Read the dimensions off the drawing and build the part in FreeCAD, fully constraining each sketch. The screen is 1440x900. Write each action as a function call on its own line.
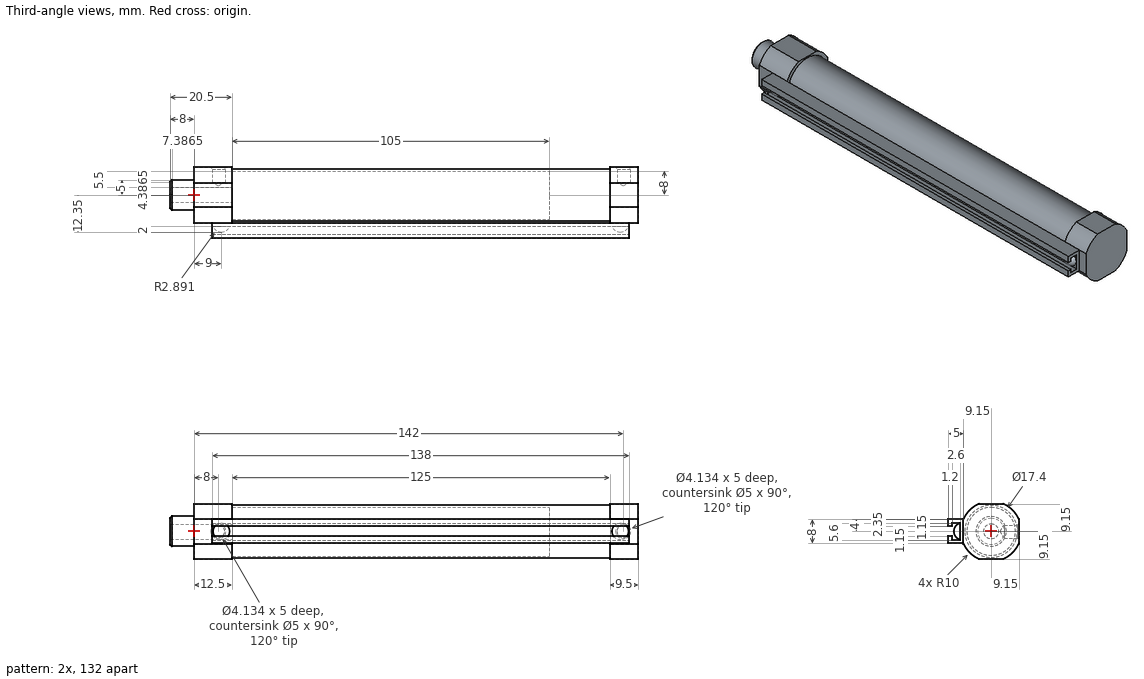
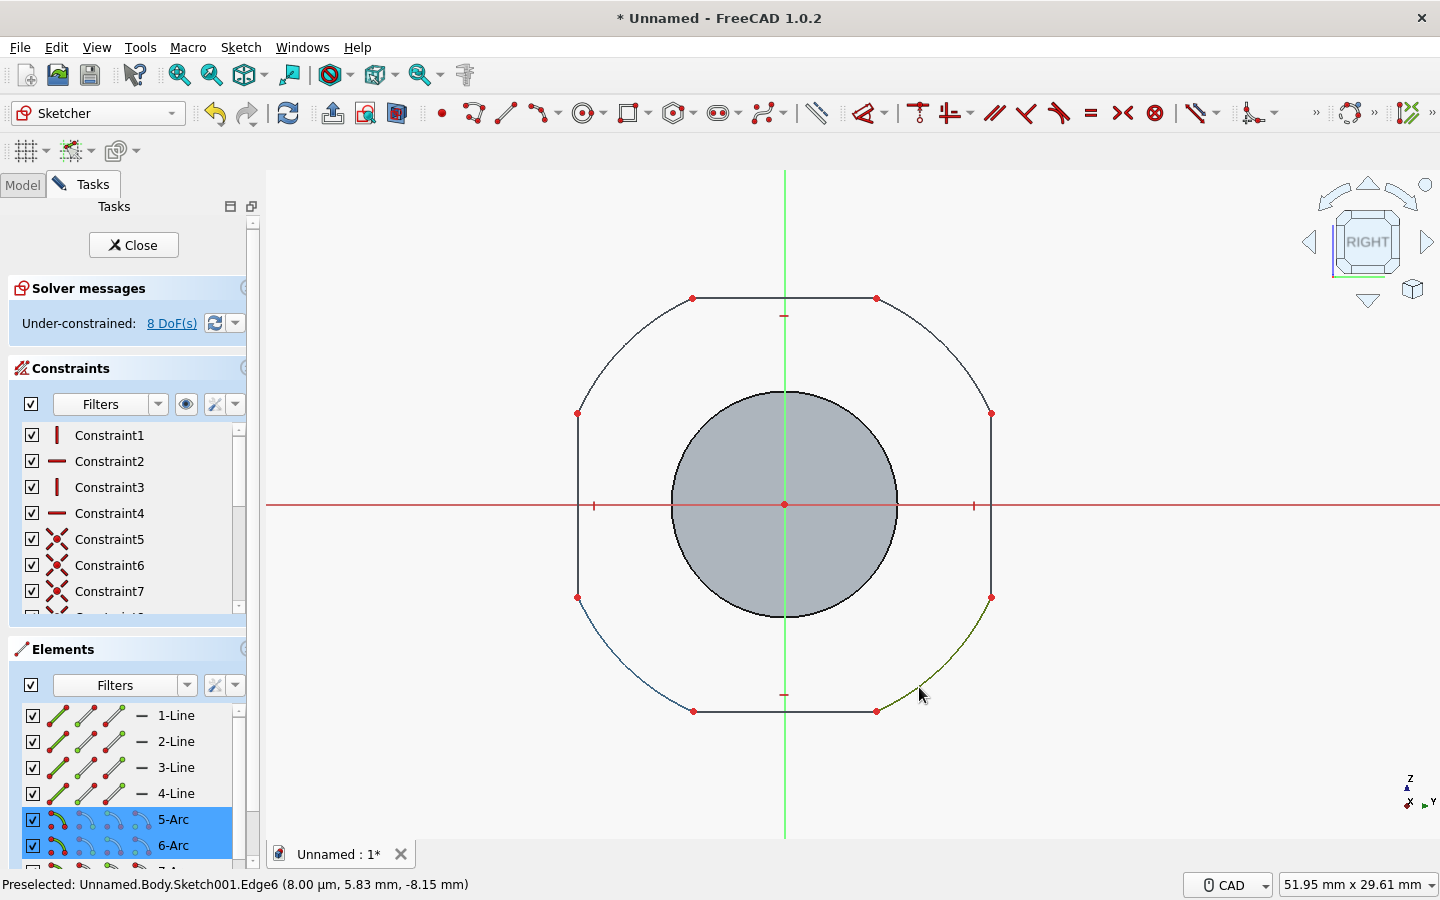
click(966, 371)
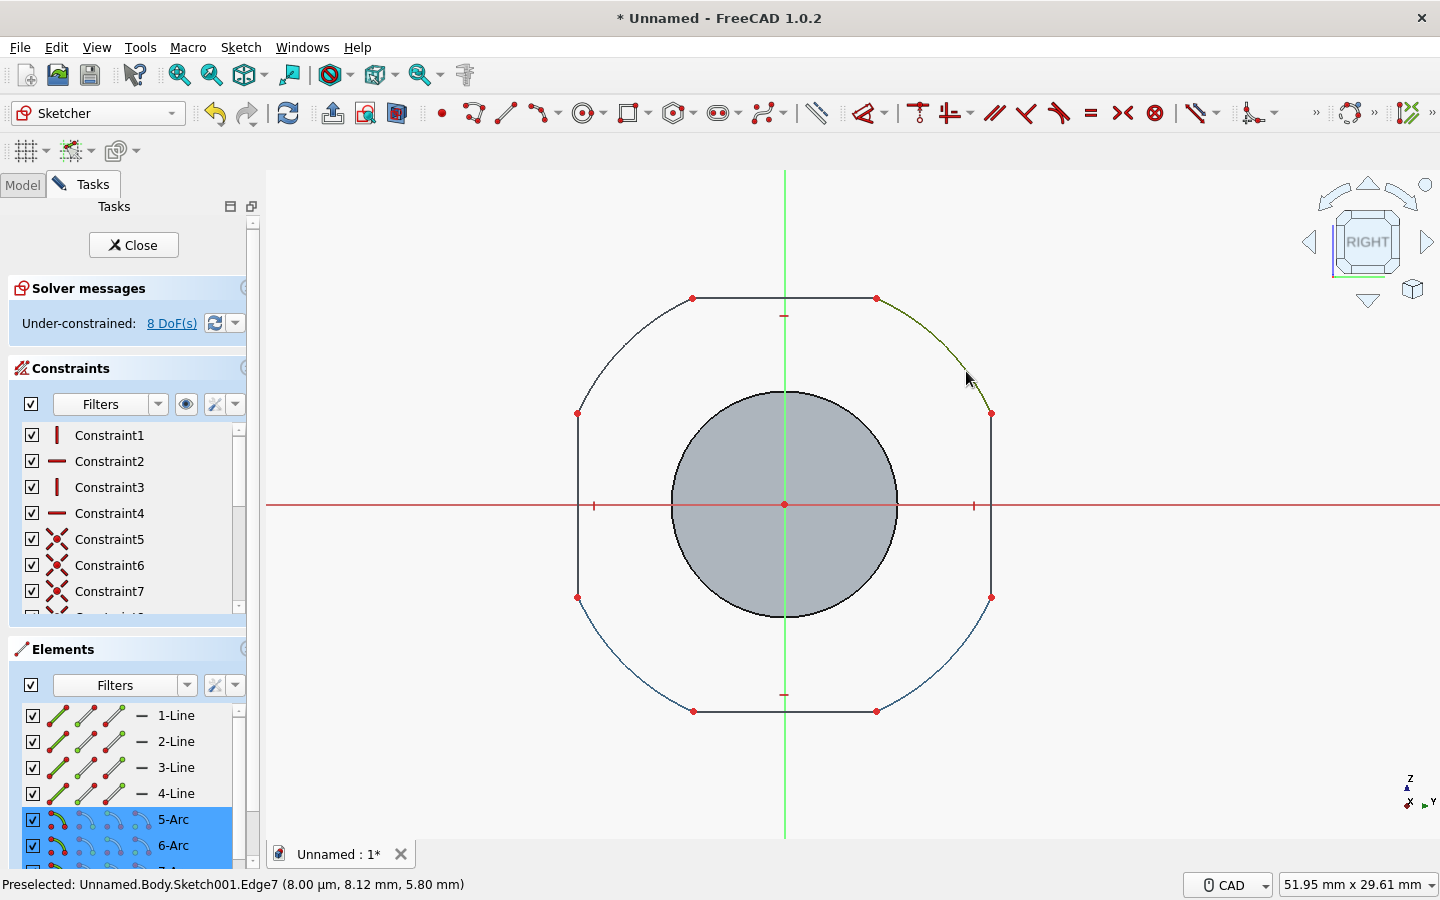
click(650, 324)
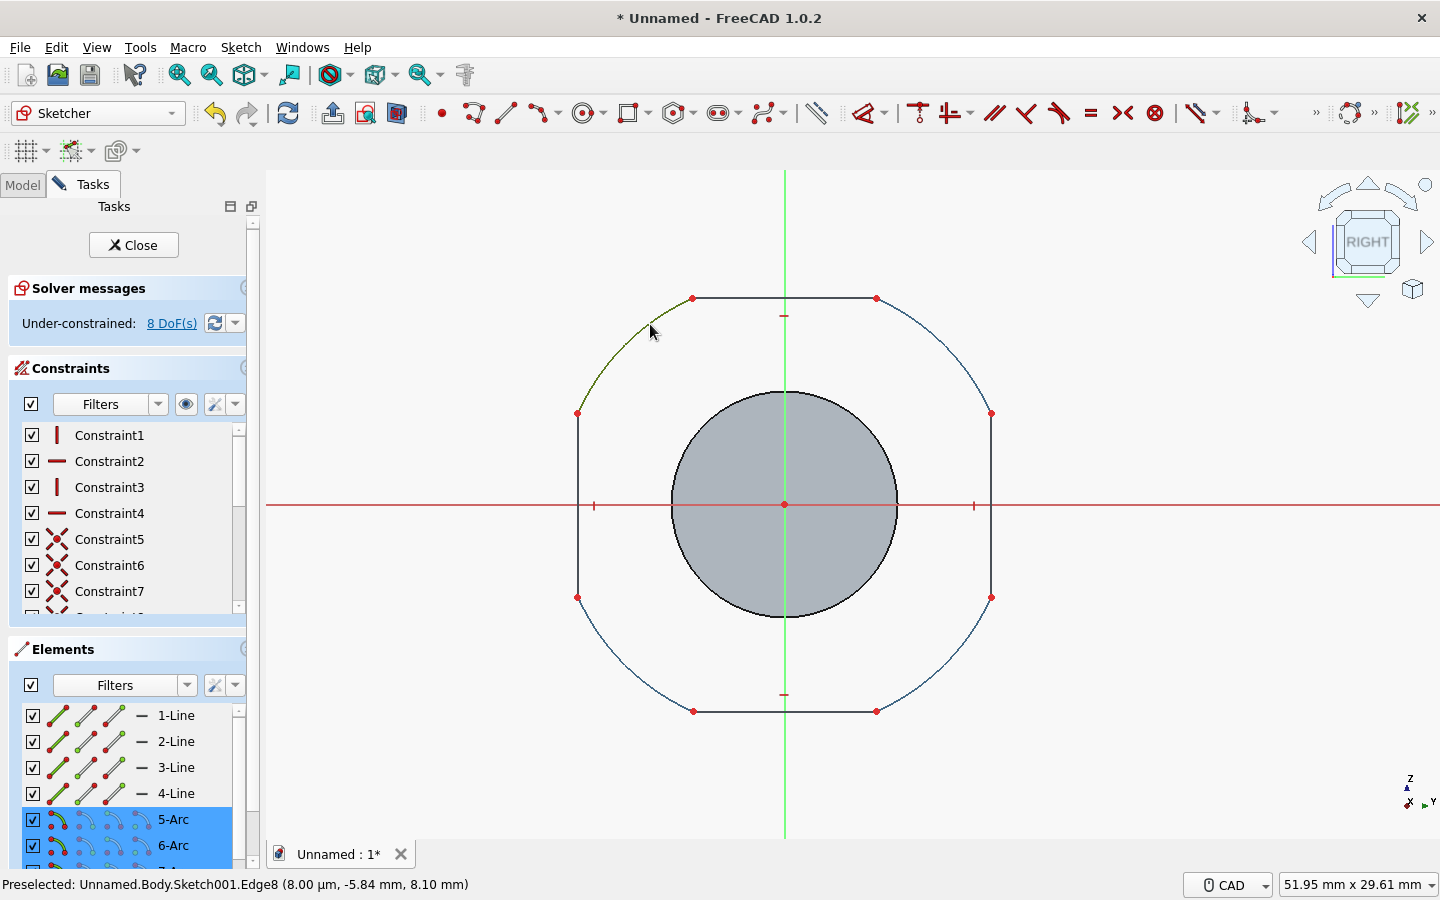
click(1092, 114)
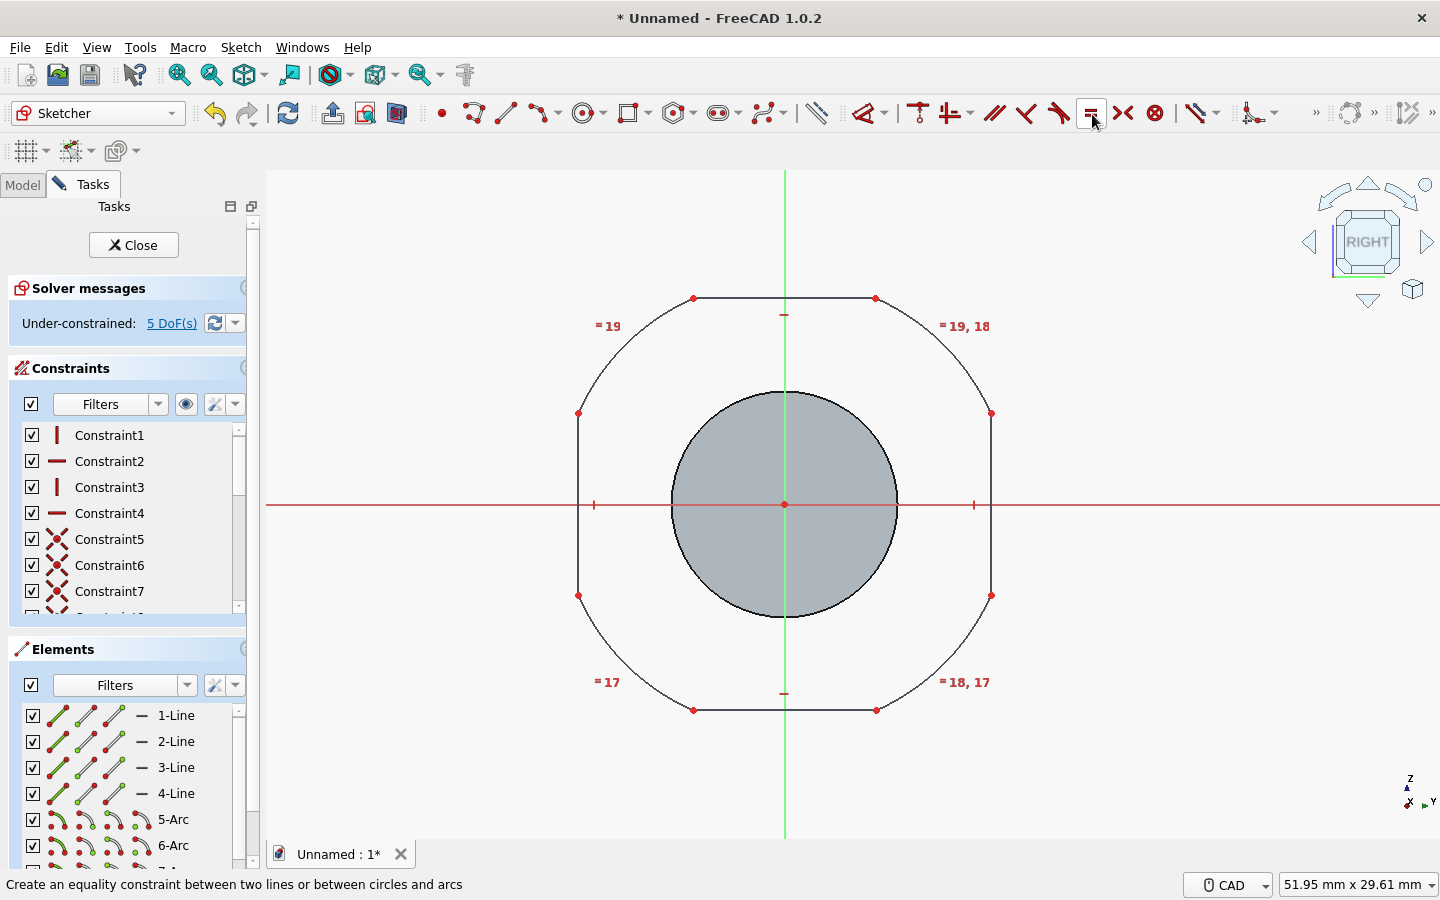
click(864, 114)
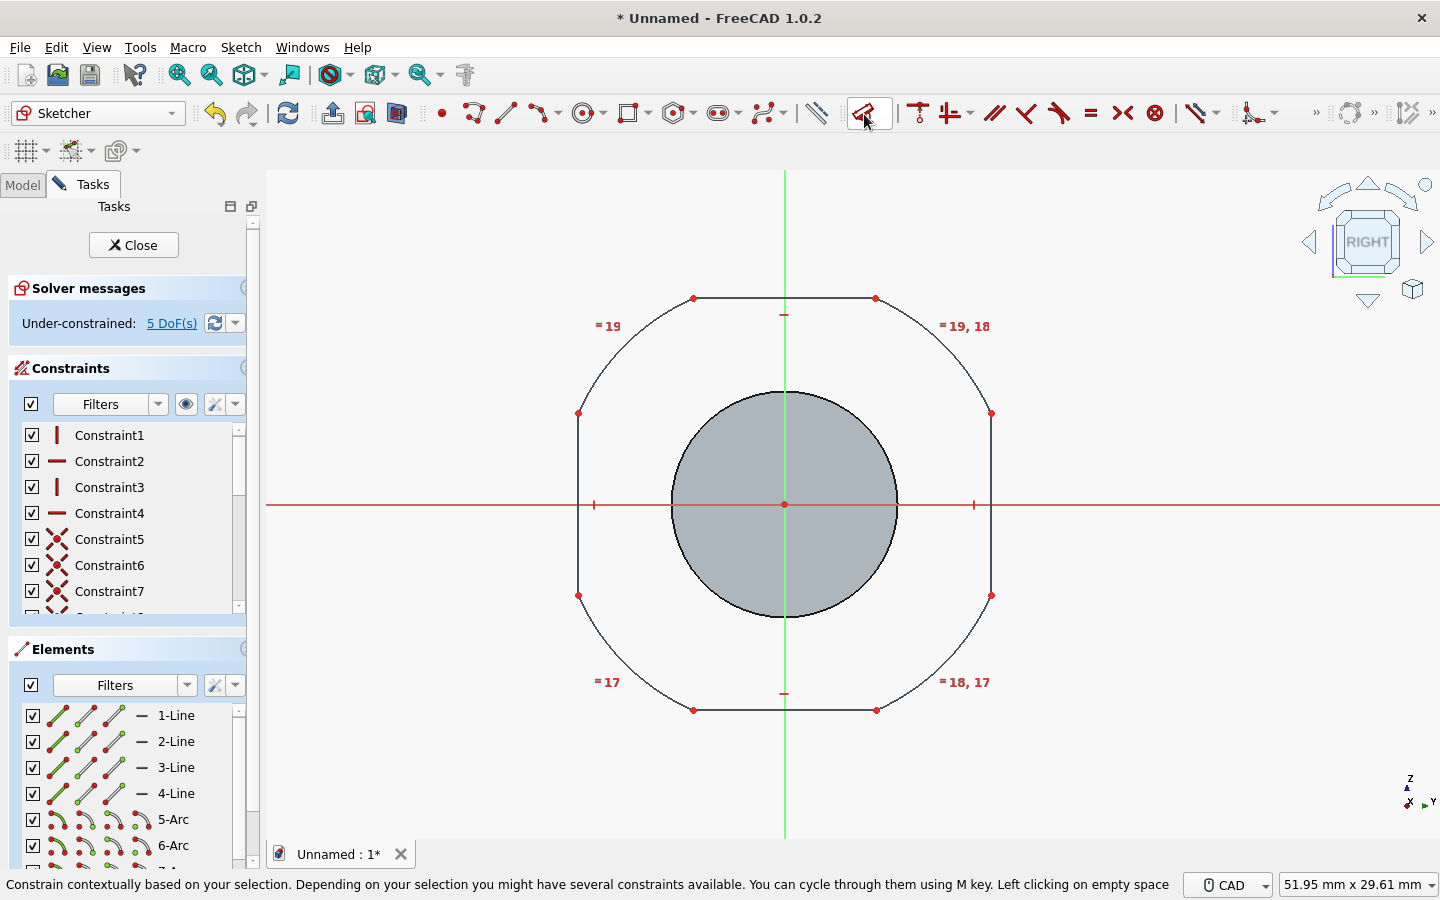
click(603, 638)
click(577, 657)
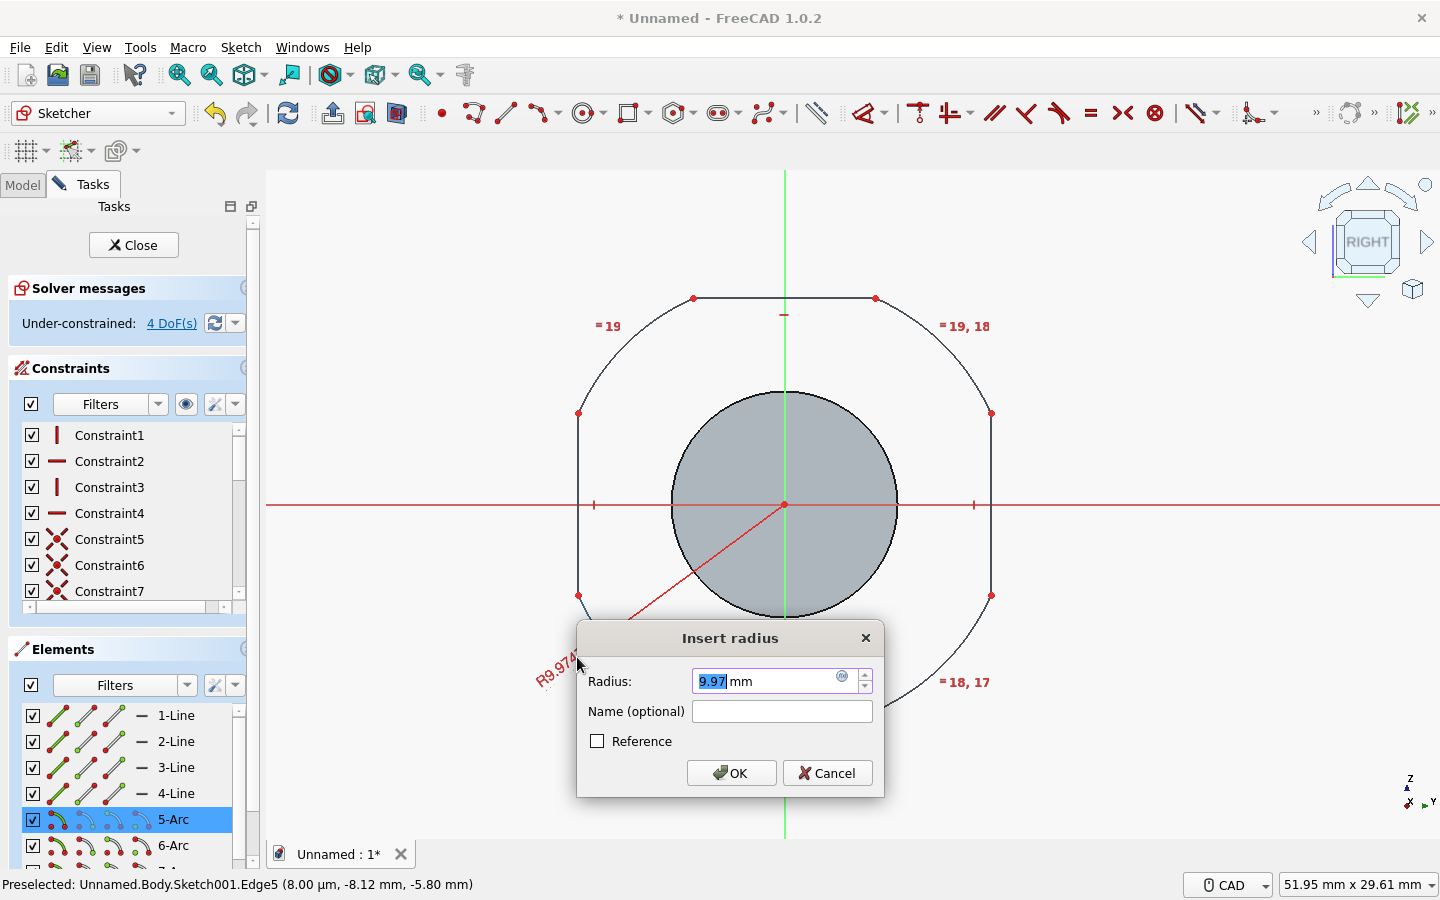
text(10)
key(Return)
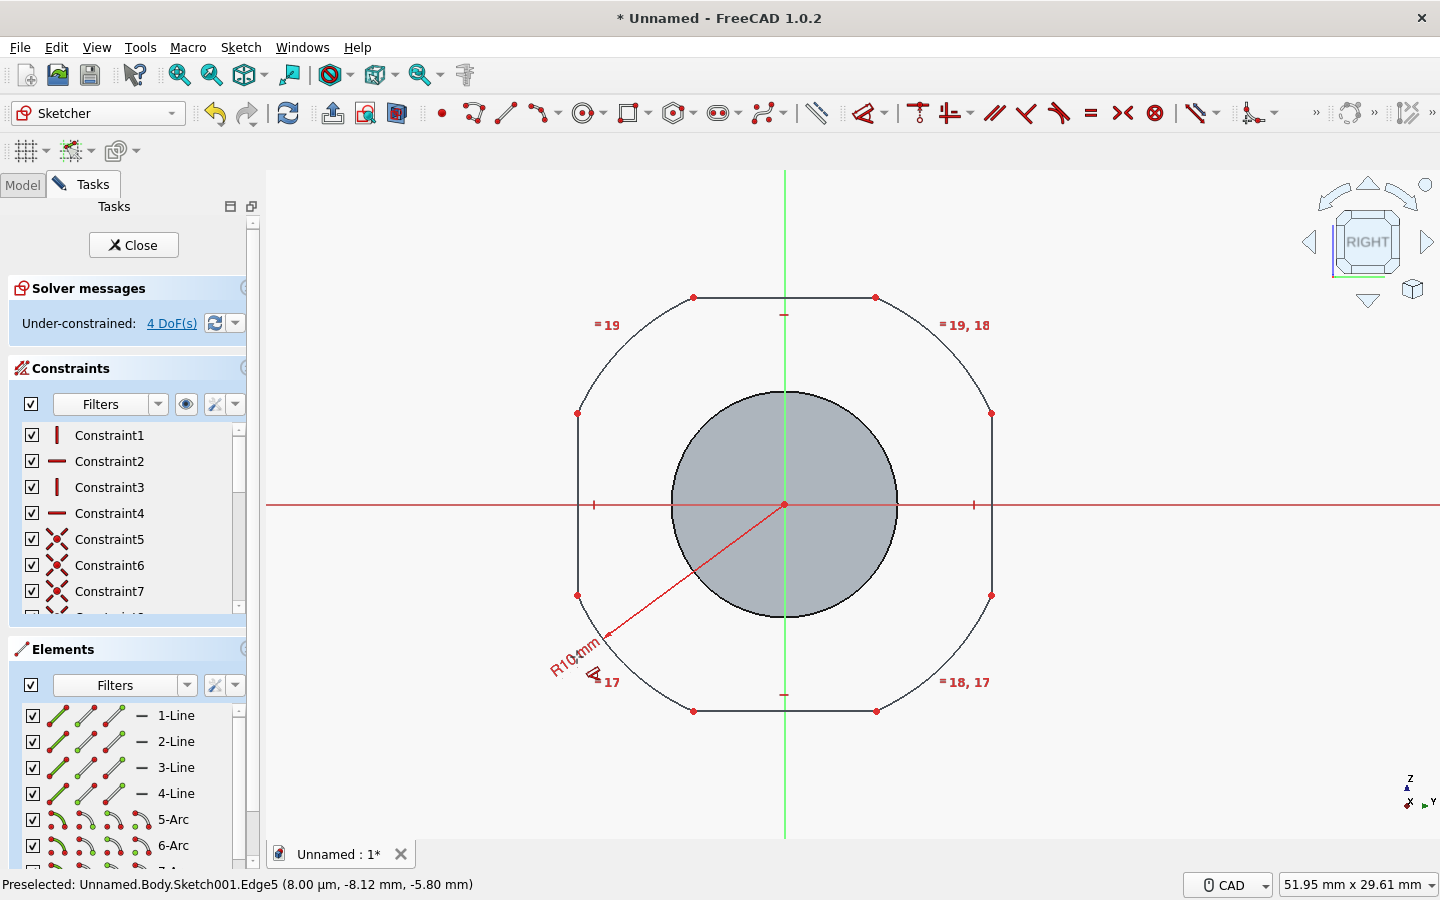
click(578, 414)
click(681, 380)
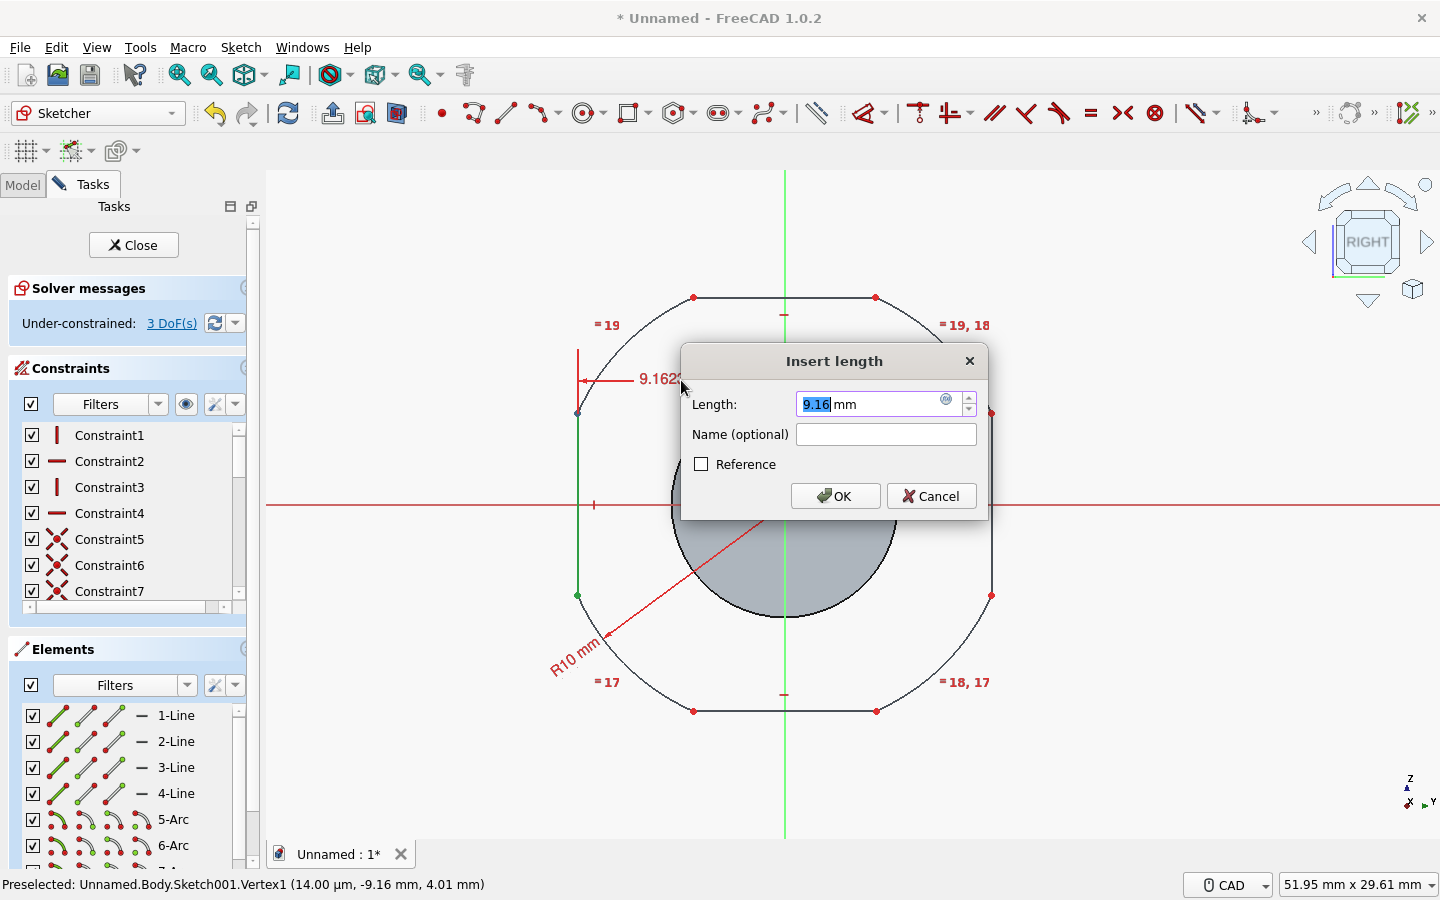
text(9.15)
key(Return)